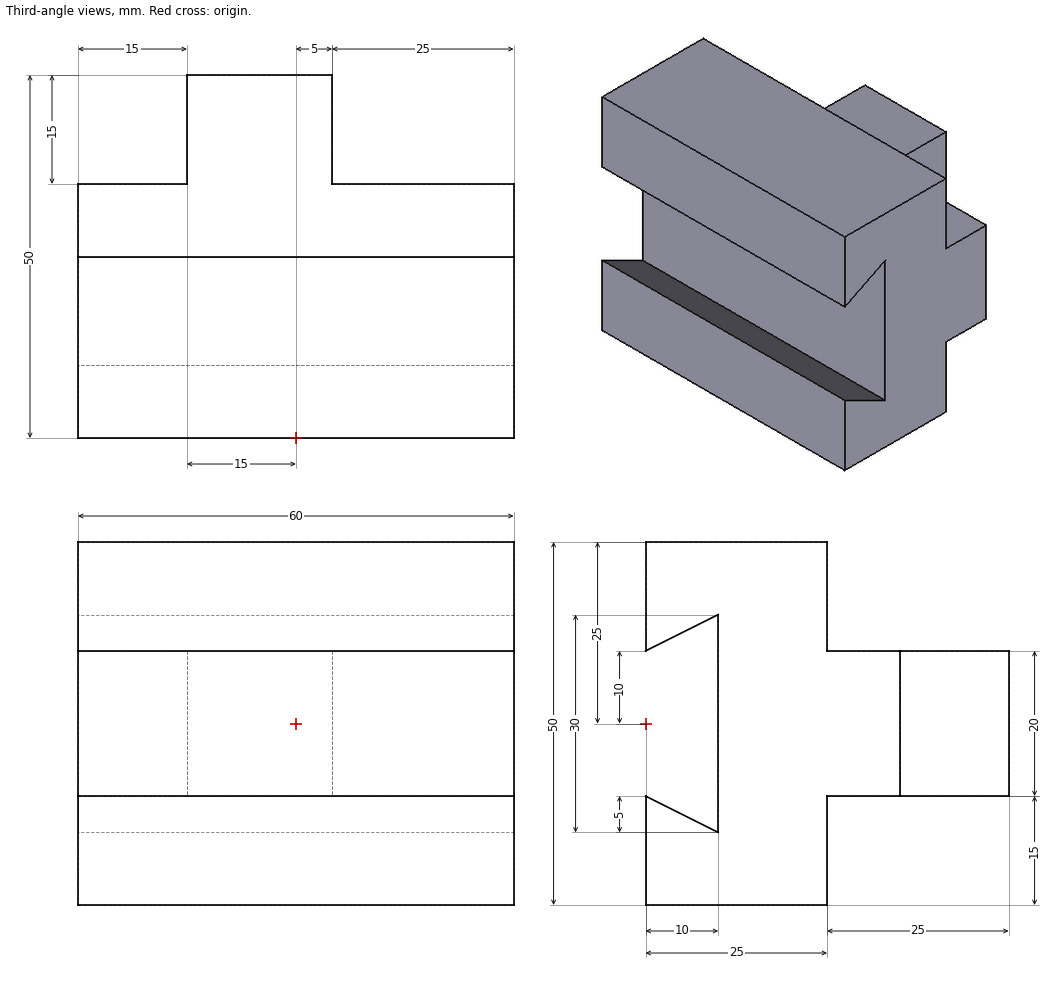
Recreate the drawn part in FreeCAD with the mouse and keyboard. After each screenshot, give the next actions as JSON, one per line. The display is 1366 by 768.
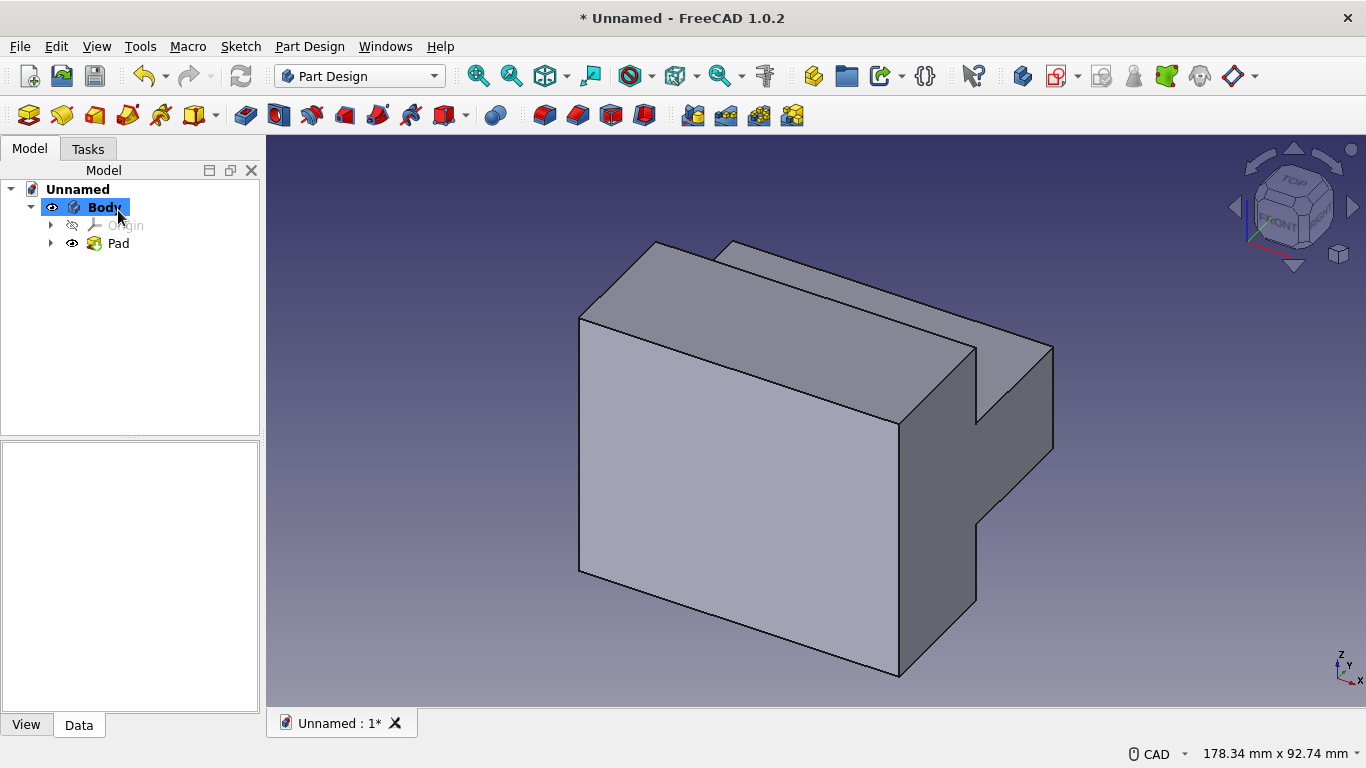
{"action": "key", "text": "0"}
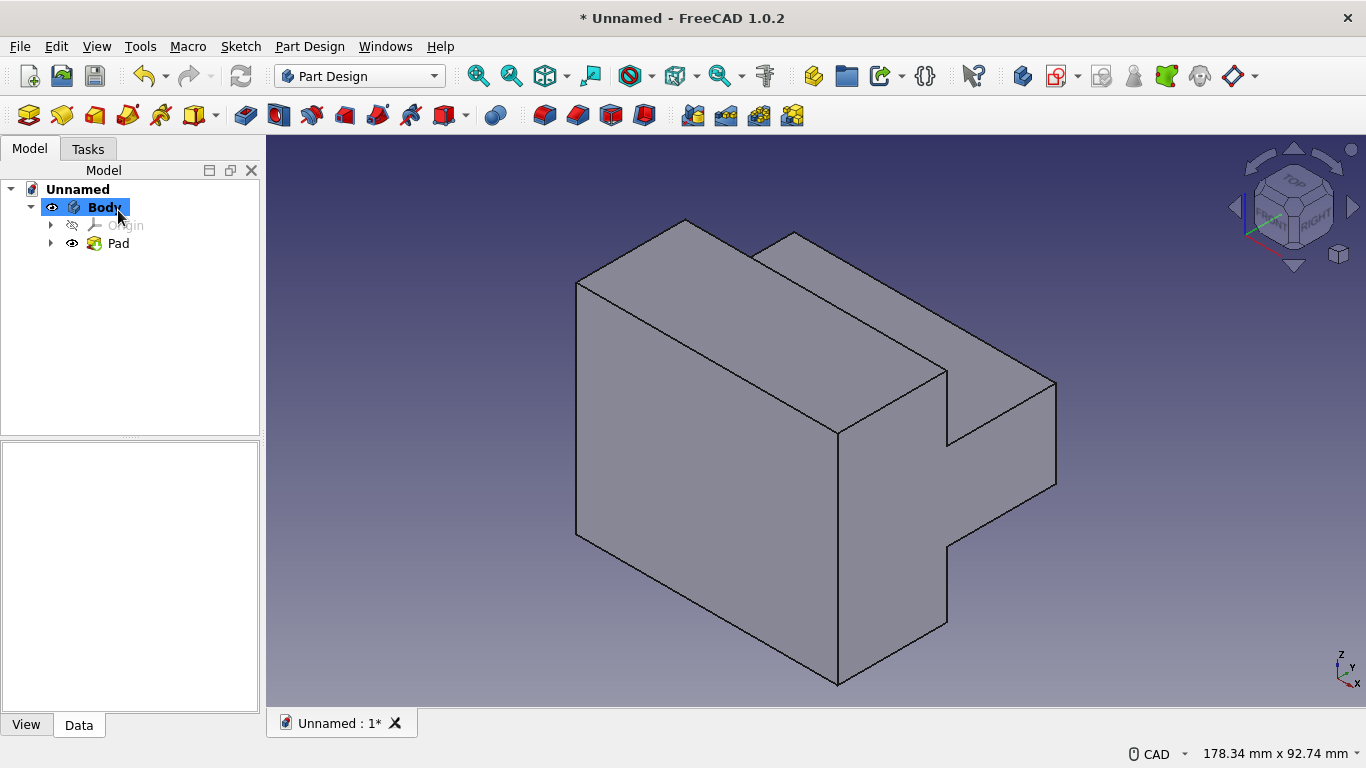
{"action": "left_click", "coordinate": [961, 372]}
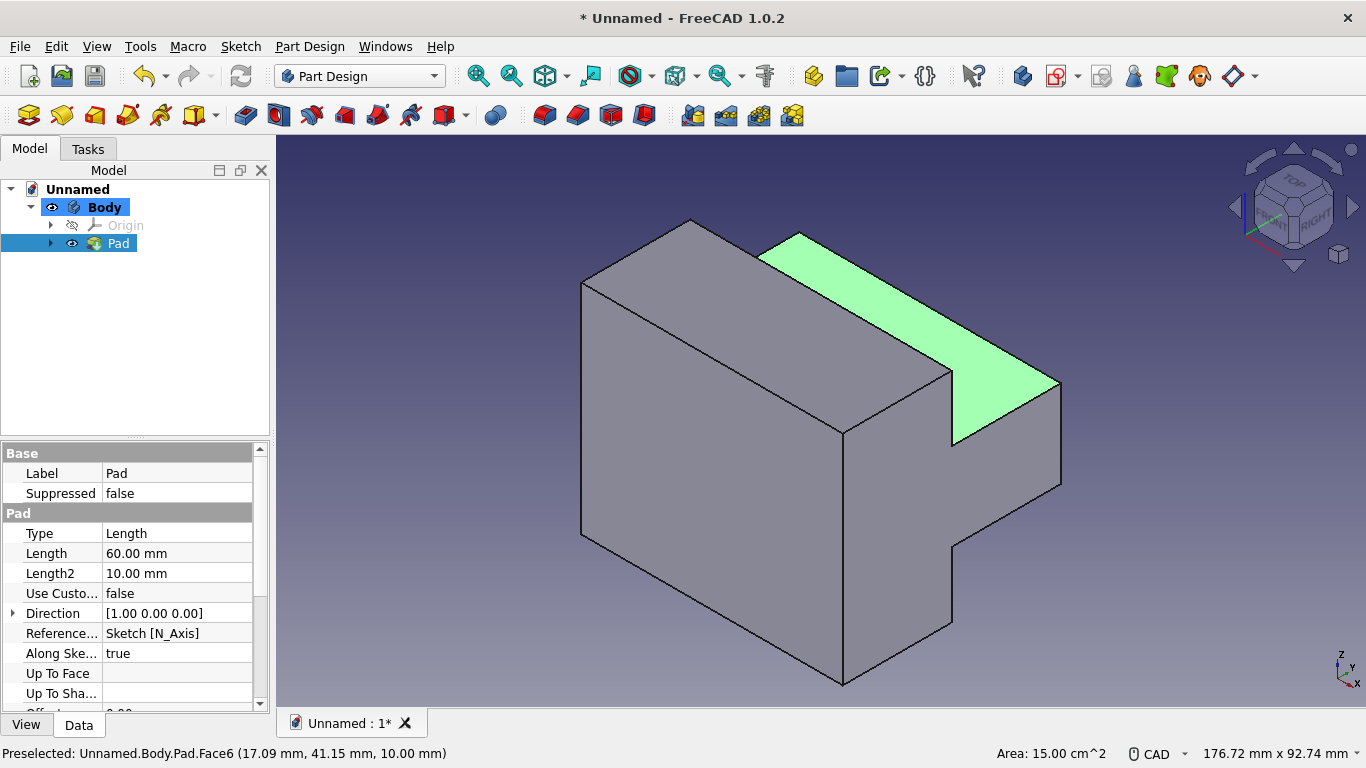
{"action": "left_click", "coordinate": [1056, 76]}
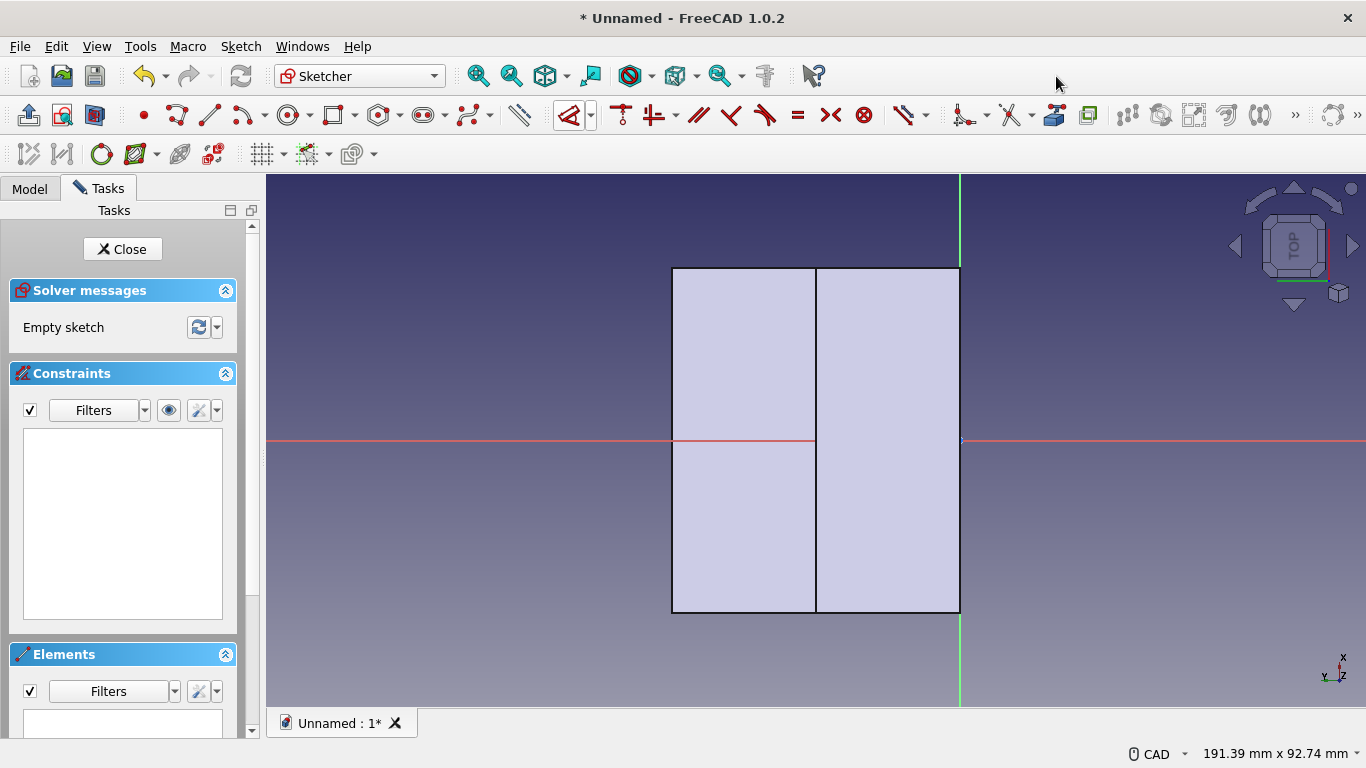
{"action": "left_click", "coordinate": [95, 116]}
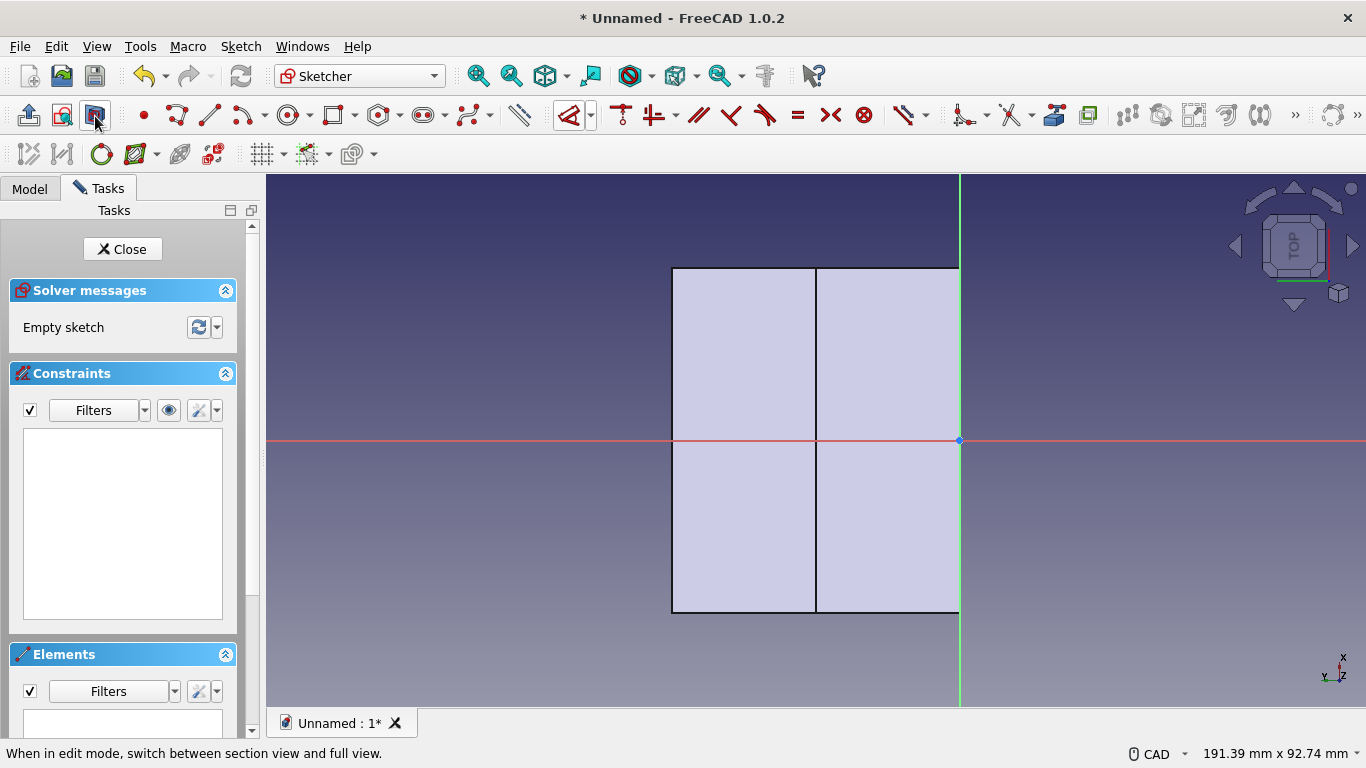
{"action": "scroll", "coordinate": [705, 612], "scroll_direction": "up", "scroll_amount": 7}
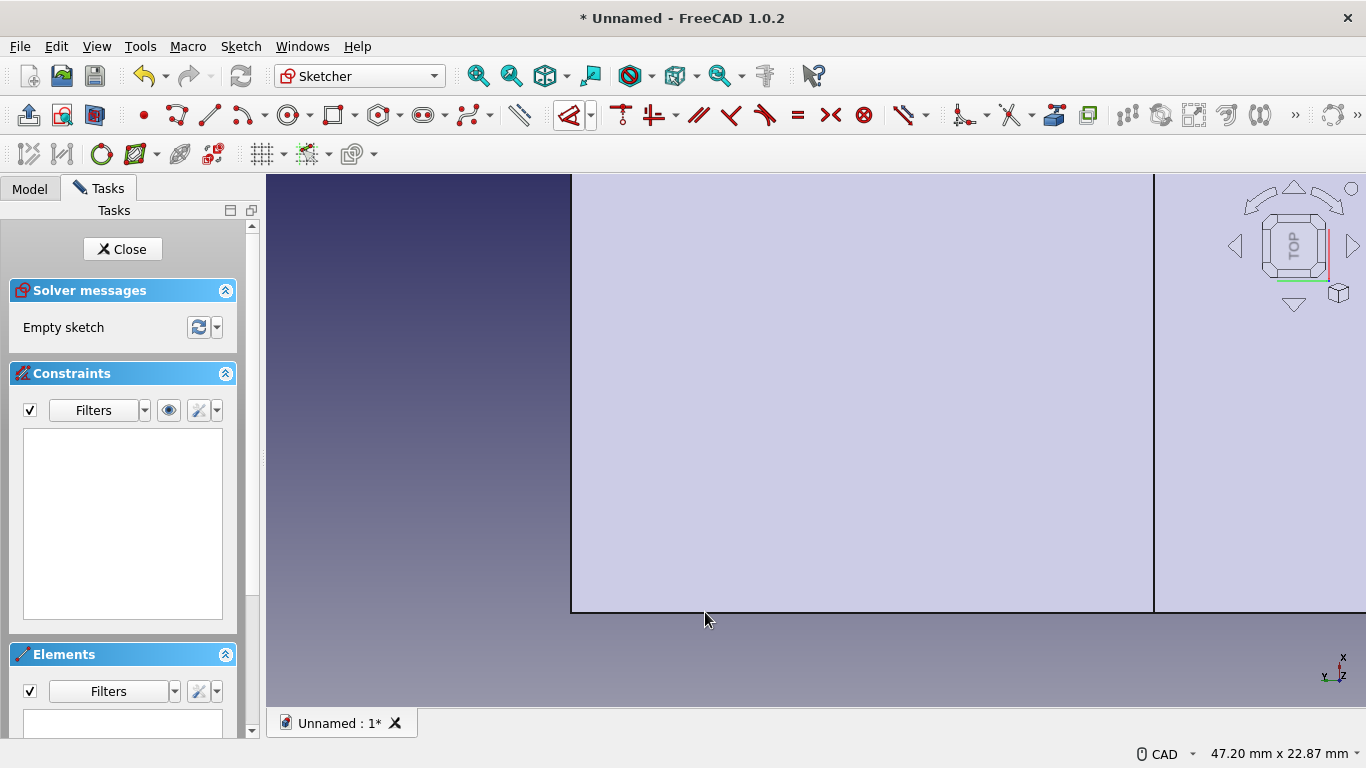
{"action": "left_click", "coordinate": [332, 116]}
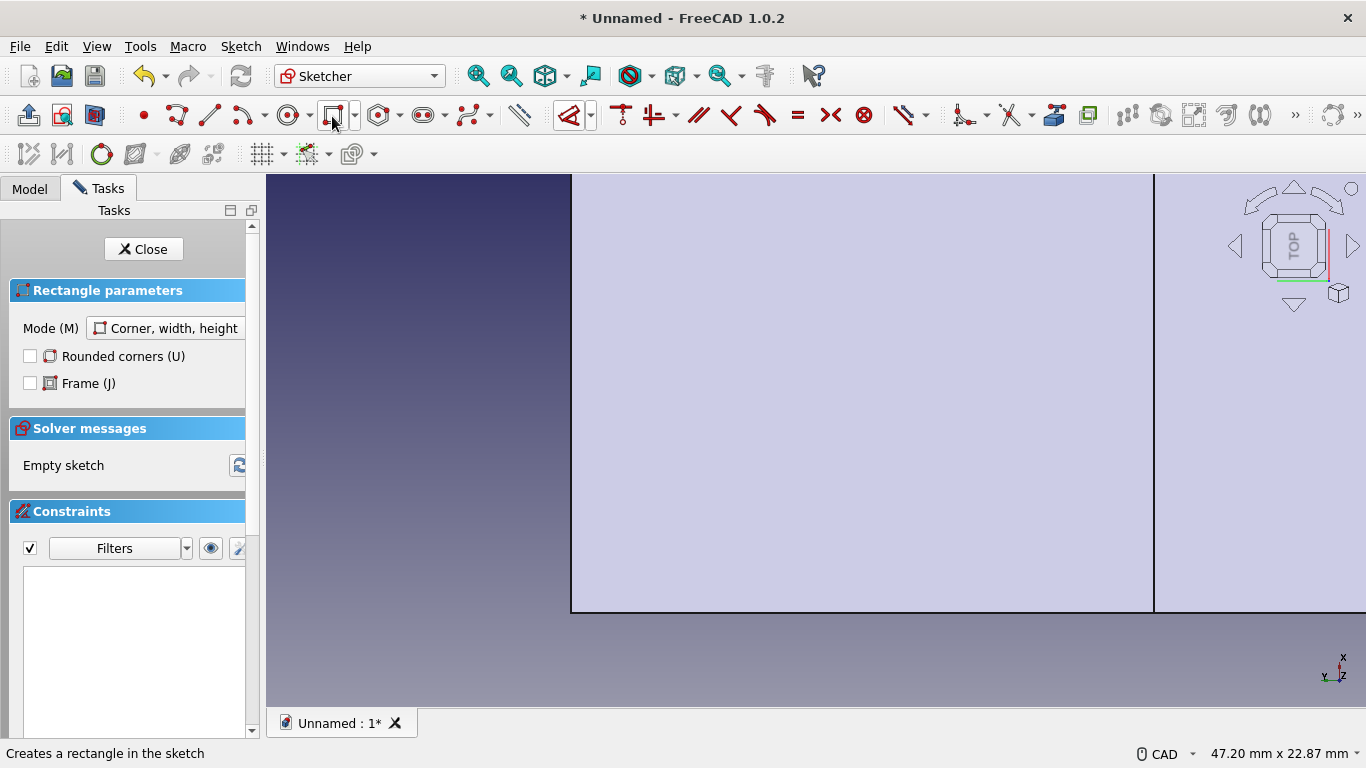
{"action": "left_click", "coordinate": [571, 264]}
{"action": "mouse_move", "coordinate": [921, 613]}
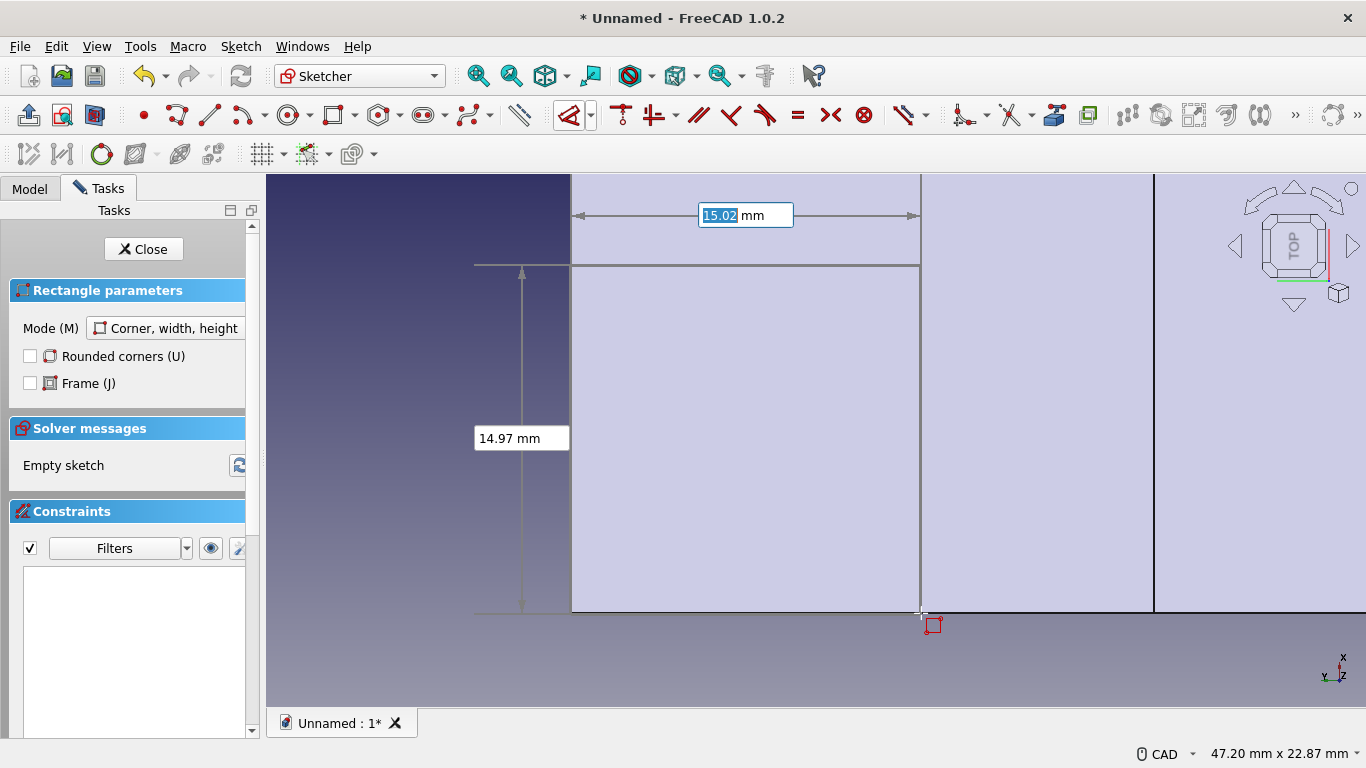
{"action": "type", "text": "15"}
{"action": "key", "text": "Tab"}
{"action": "type", "text": "15"}
{"action": "key", "text": "Return"}
{"action": "key", "text": "Escape"}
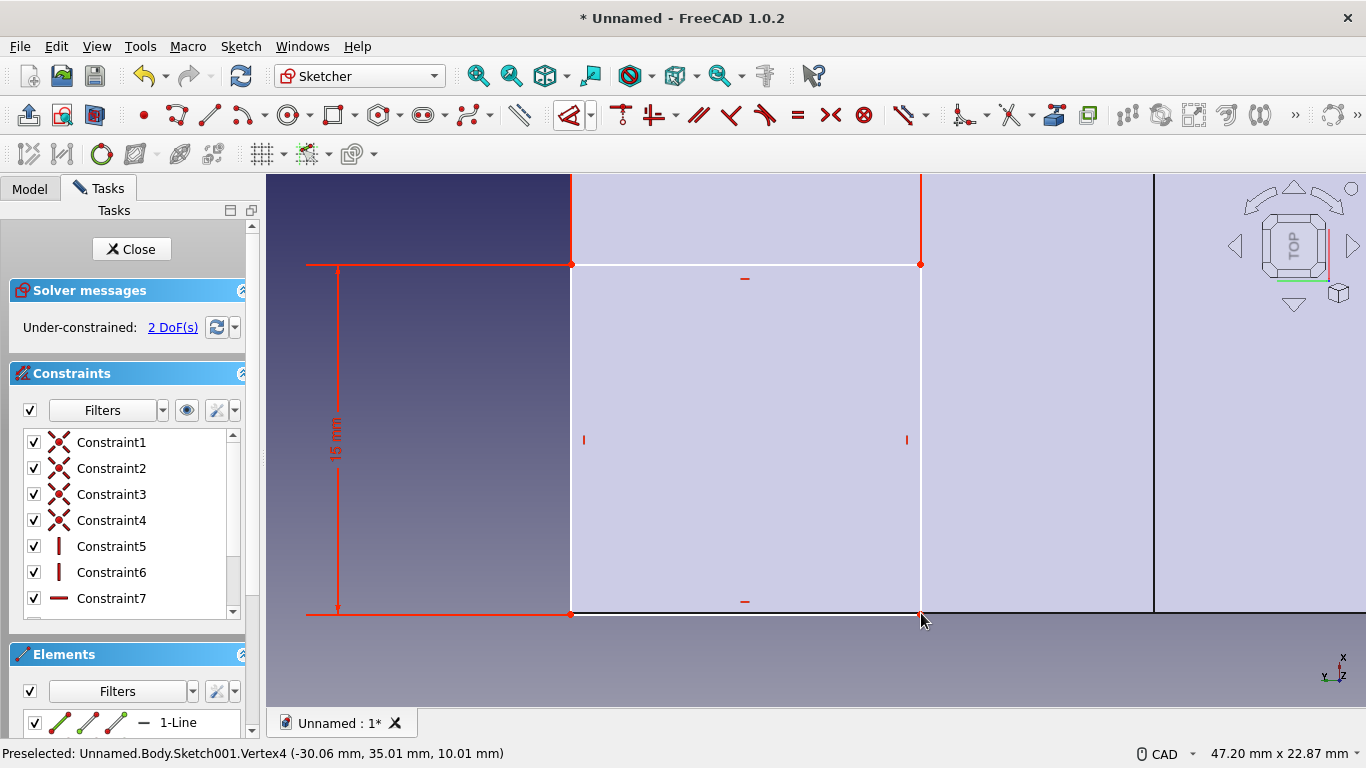
{"action": "left_click", "coordinate": [571, 265]}